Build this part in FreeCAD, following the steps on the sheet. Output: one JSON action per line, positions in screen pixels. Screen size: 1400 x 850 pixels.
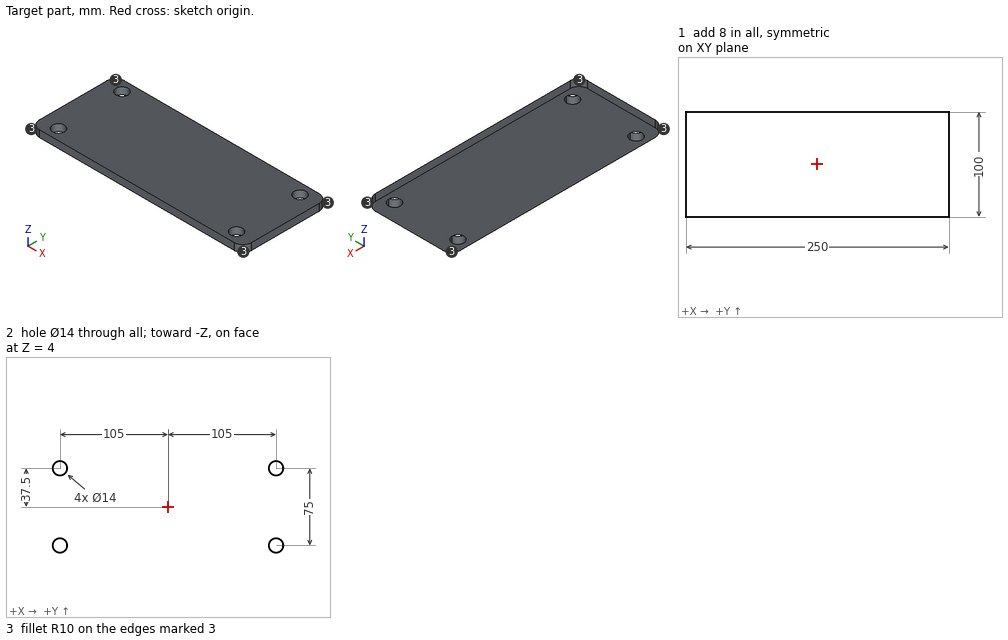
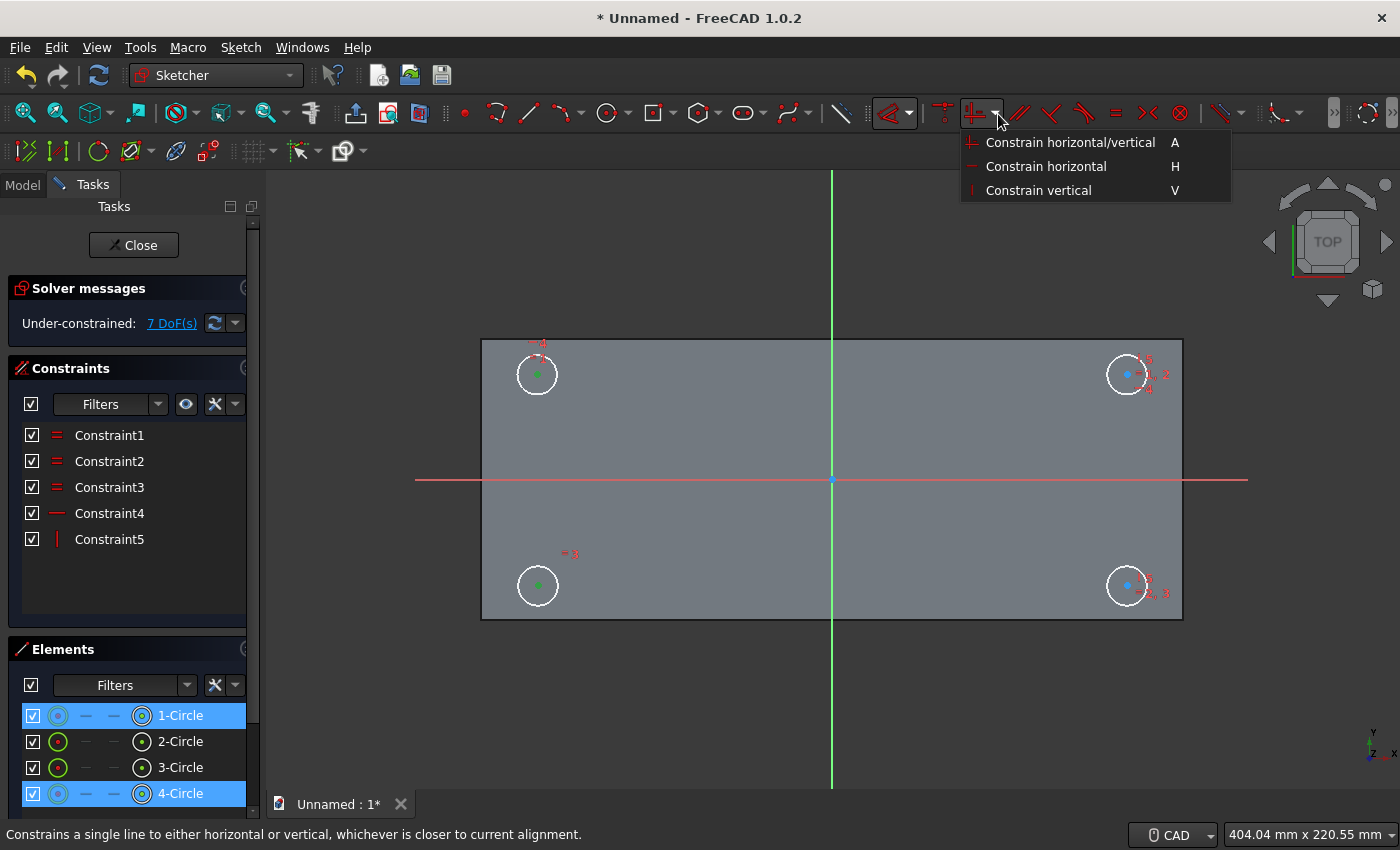
{"action": "left_click", "coordinate": [1096, 190]}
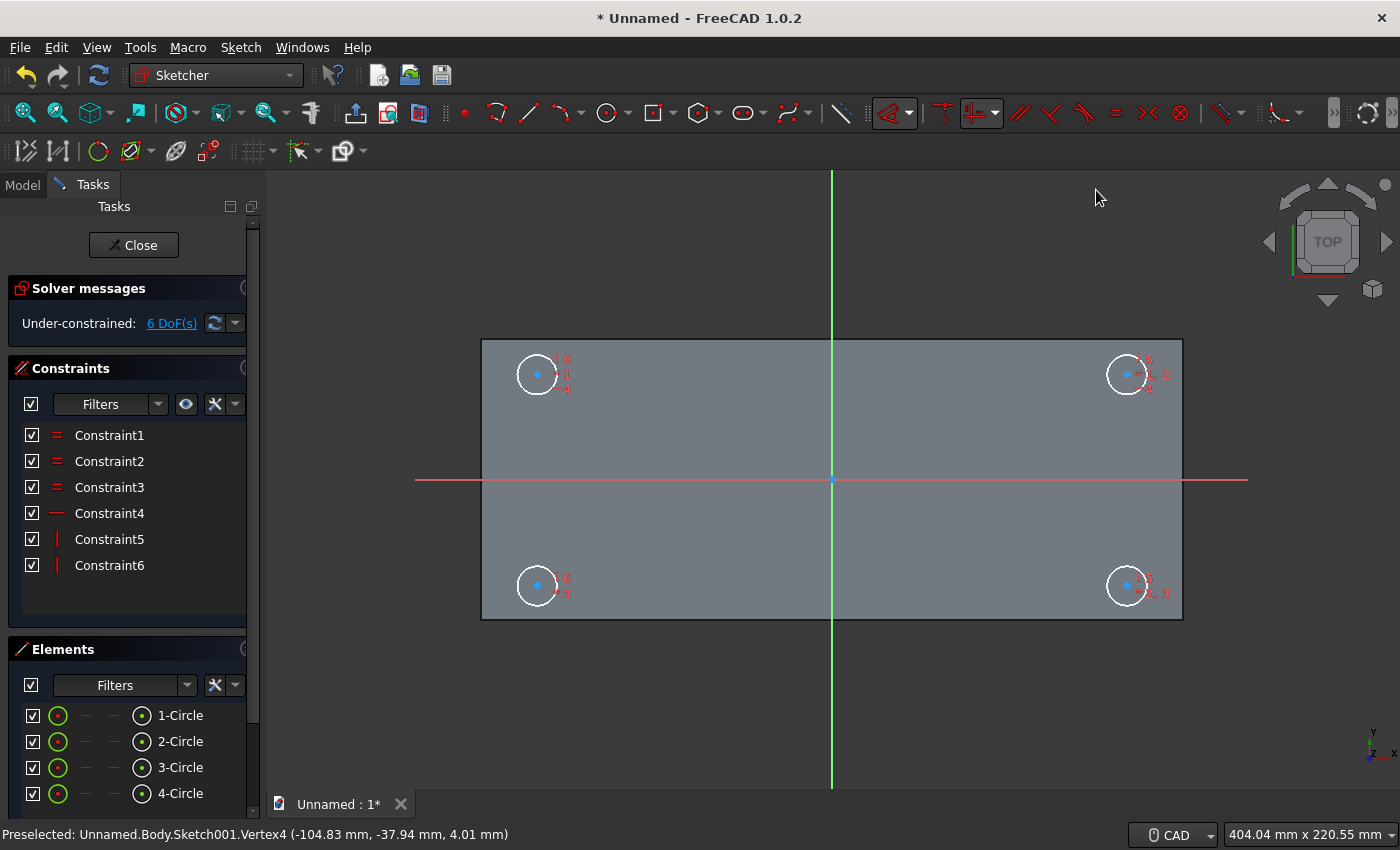
{"action": "left_click", "coordinate": [1127, 586]}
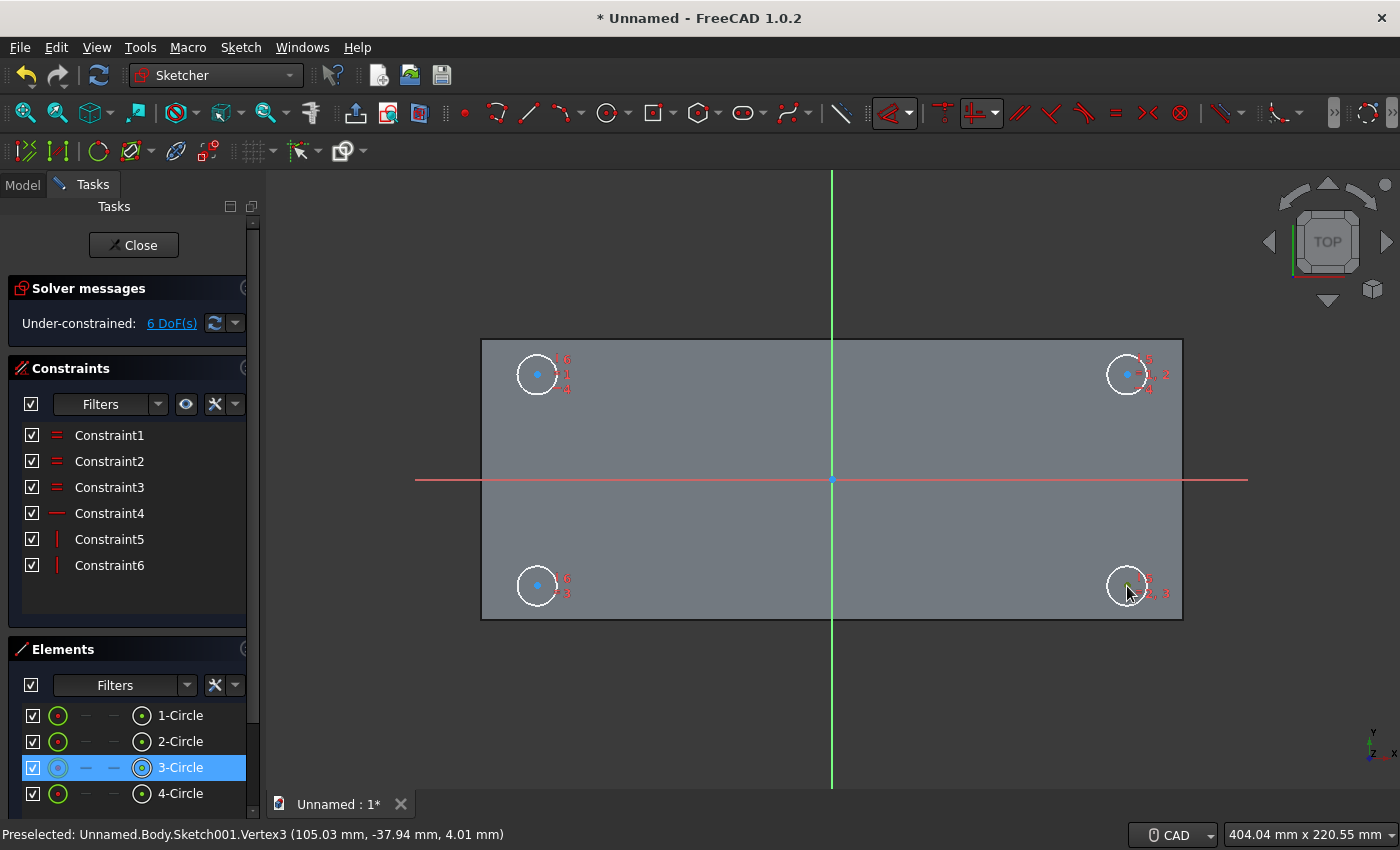
{"action": "left_click", "coordinate": [537, 586]}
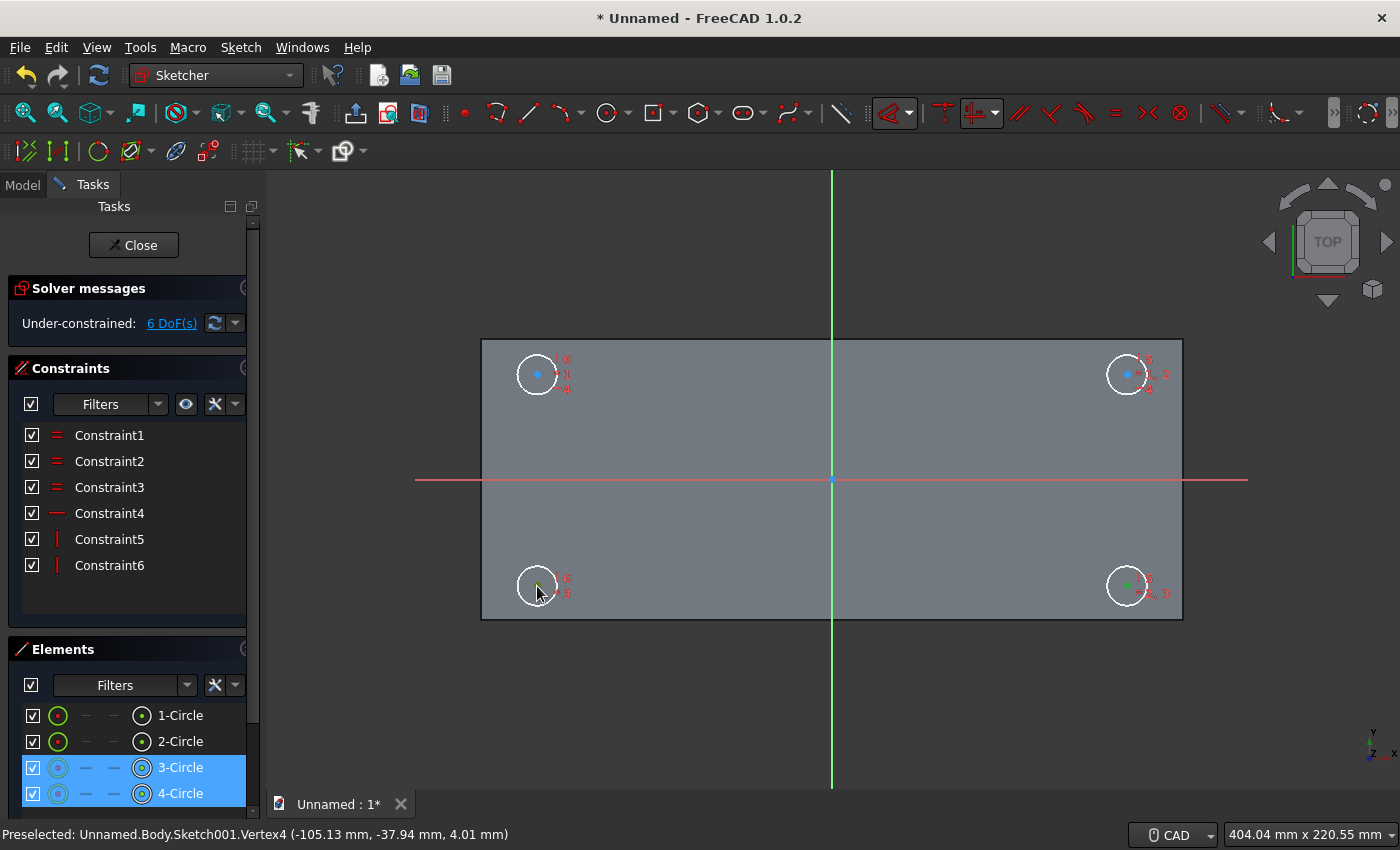
{"action": "left_click", "coordinate": [998, 114]}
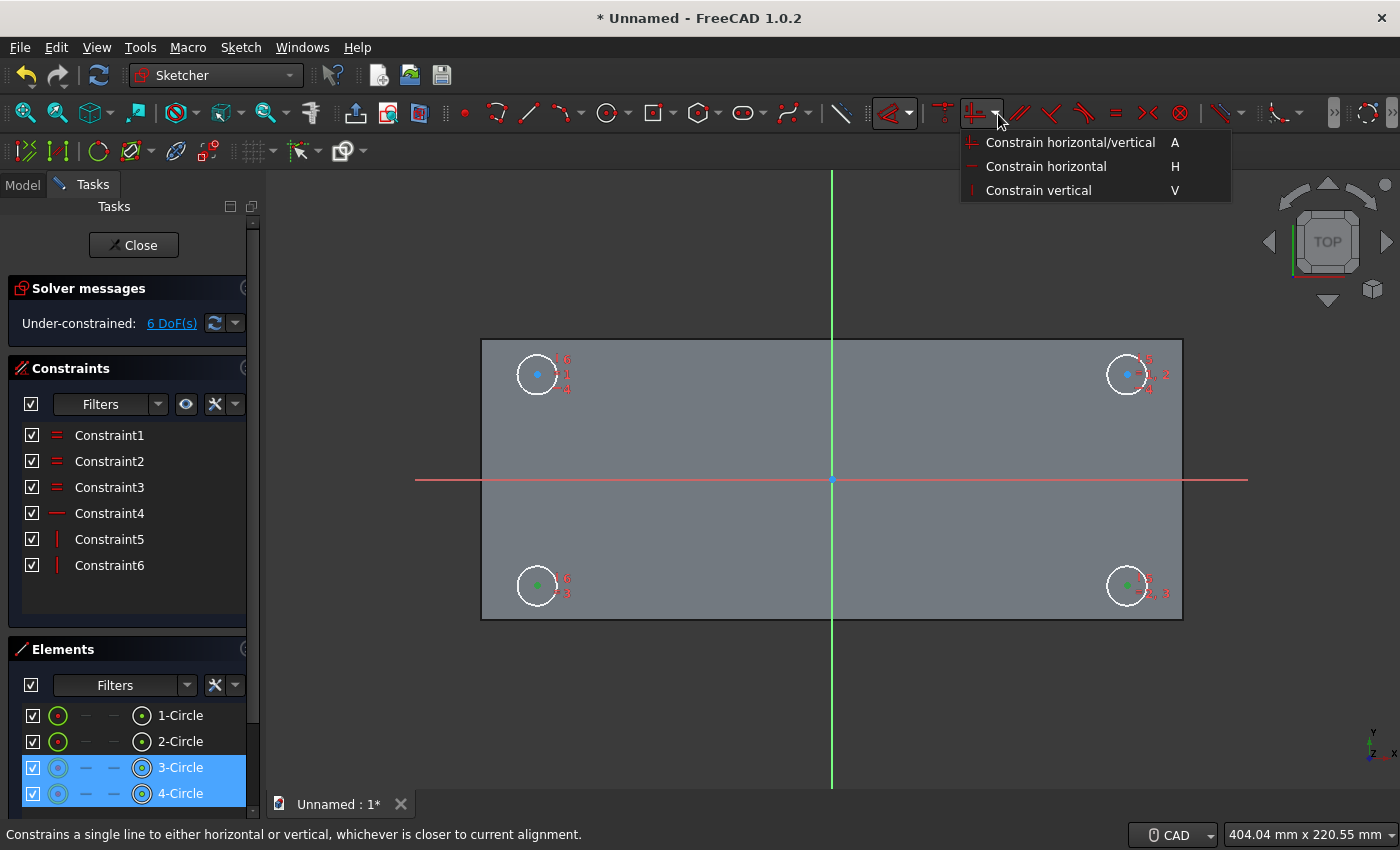
{"action": "left_click", "coordinate": [1096, 166]}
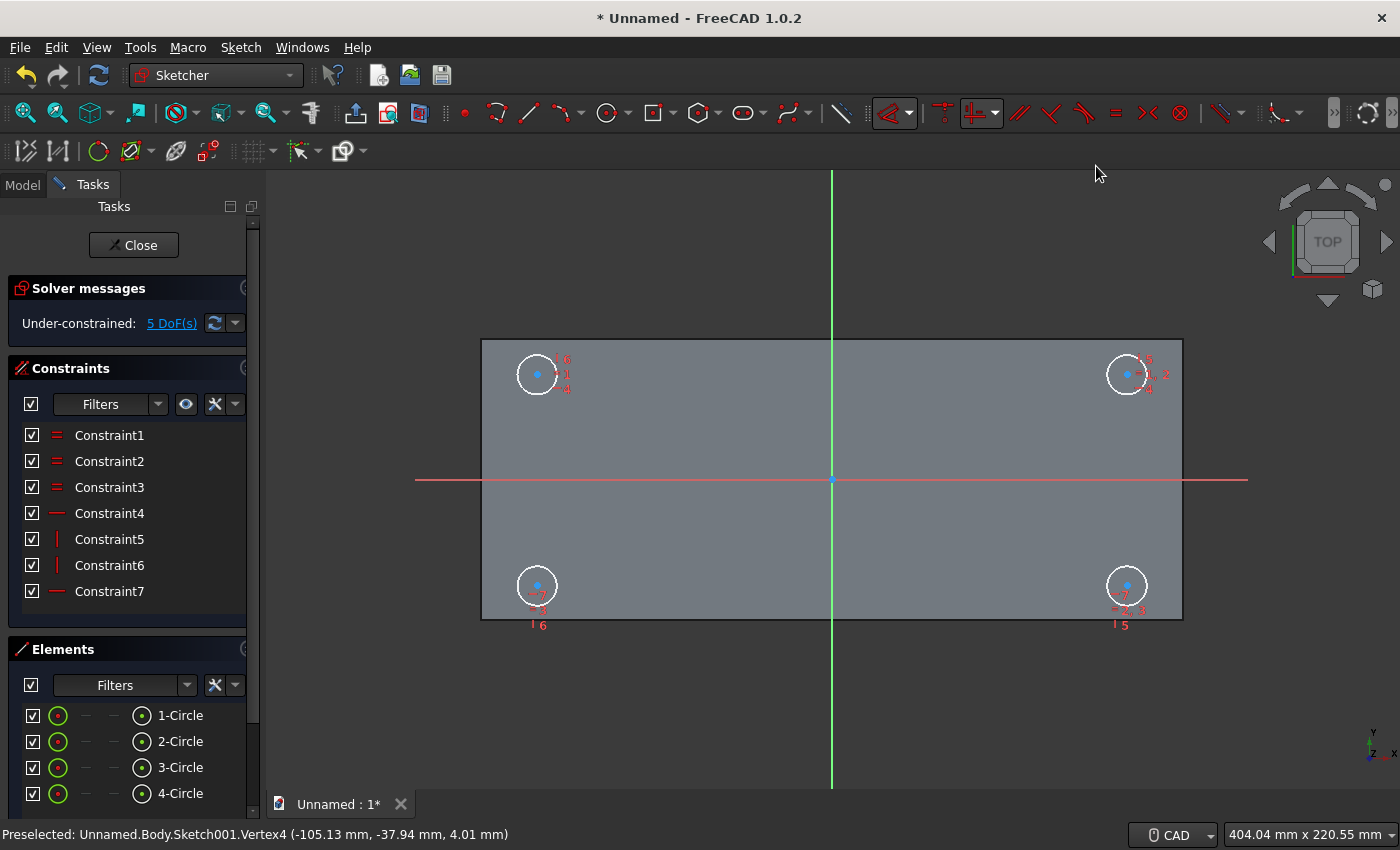
{"action": "left_click", "coordinate": [551, 361]}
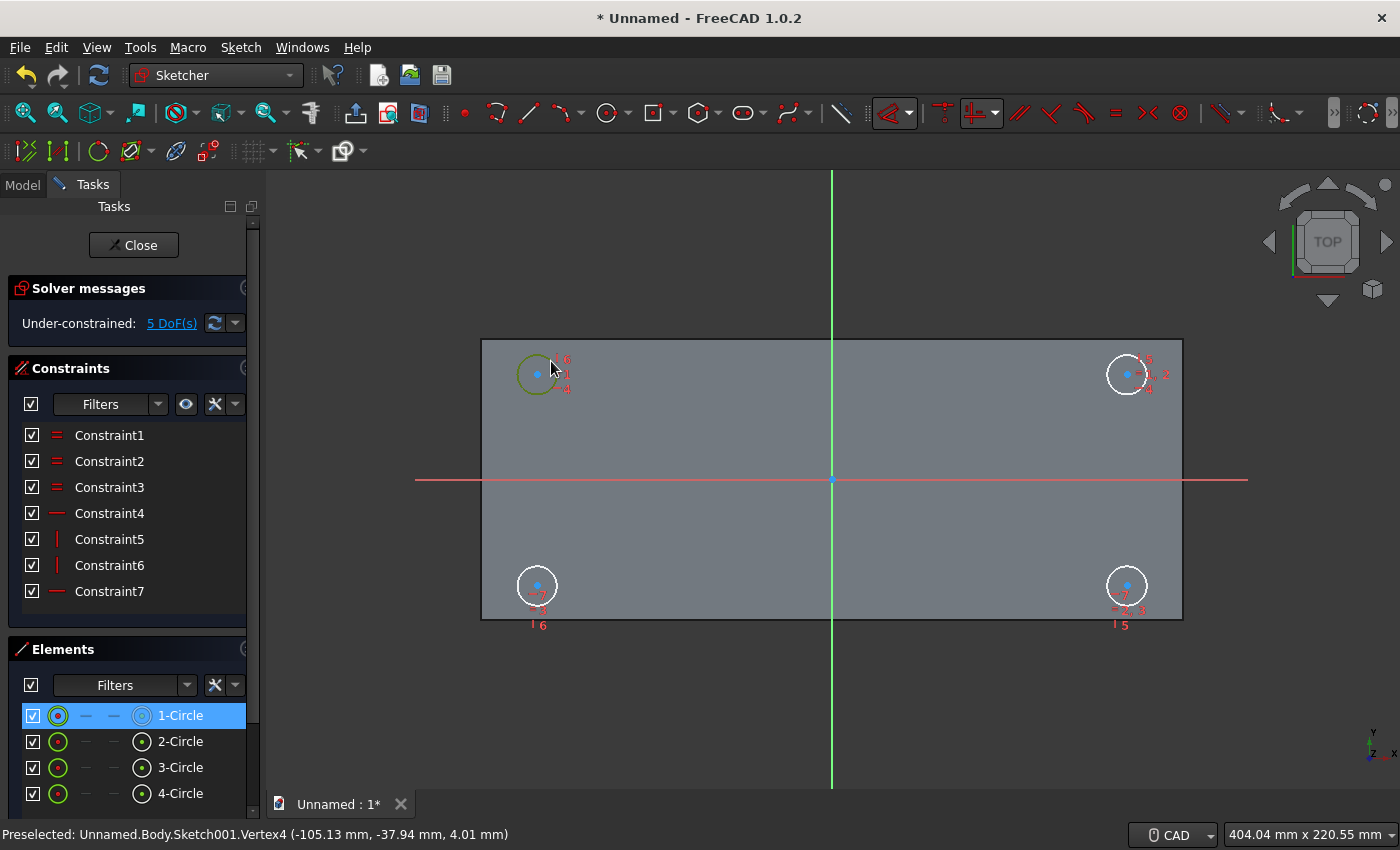
{"action": "key", "text": "k o"}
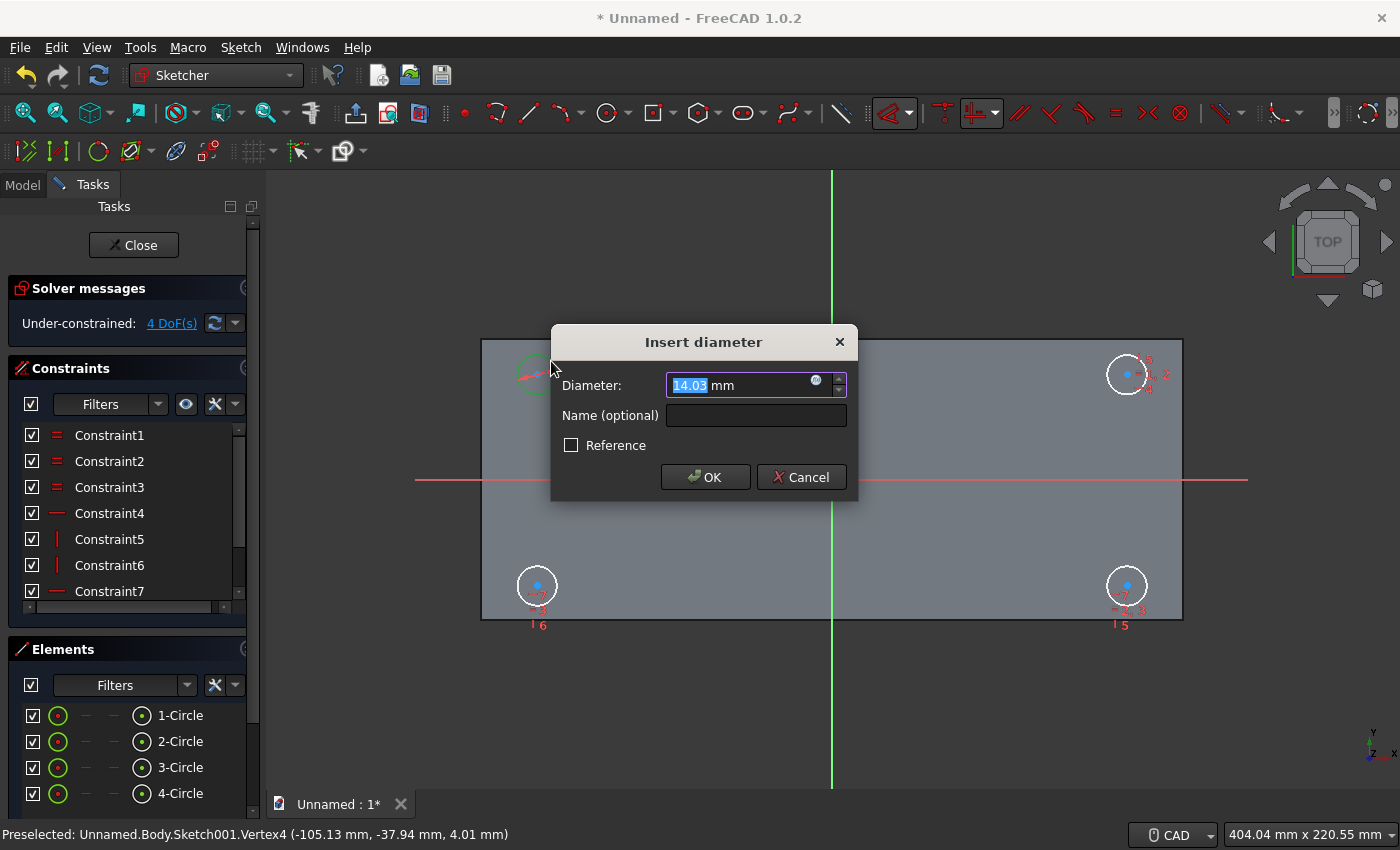
{"action": "type", "text": "14"}
{"action": "key", "text": "Return"}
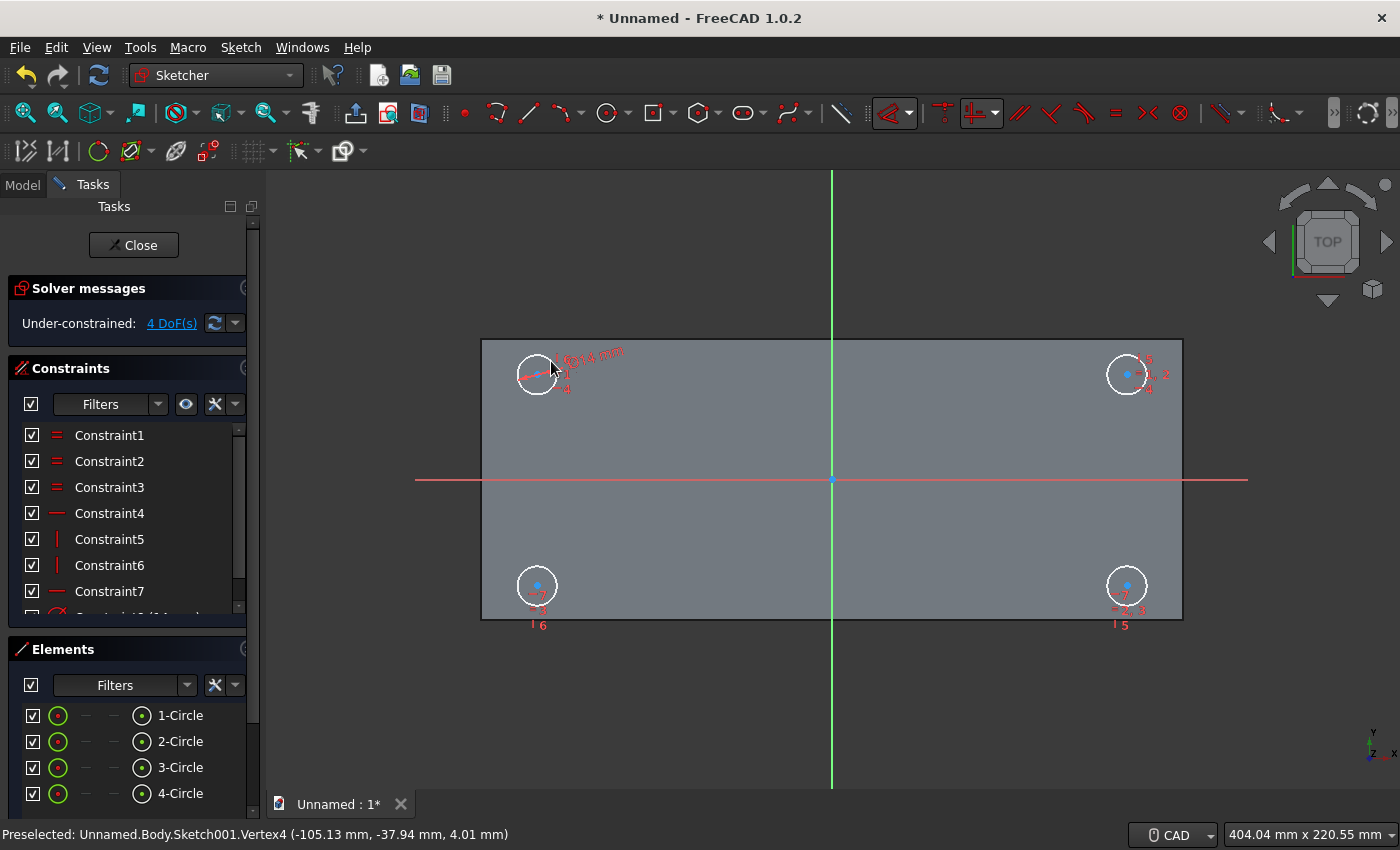
{"action": "left_click", "coordinate": [537, 375]}